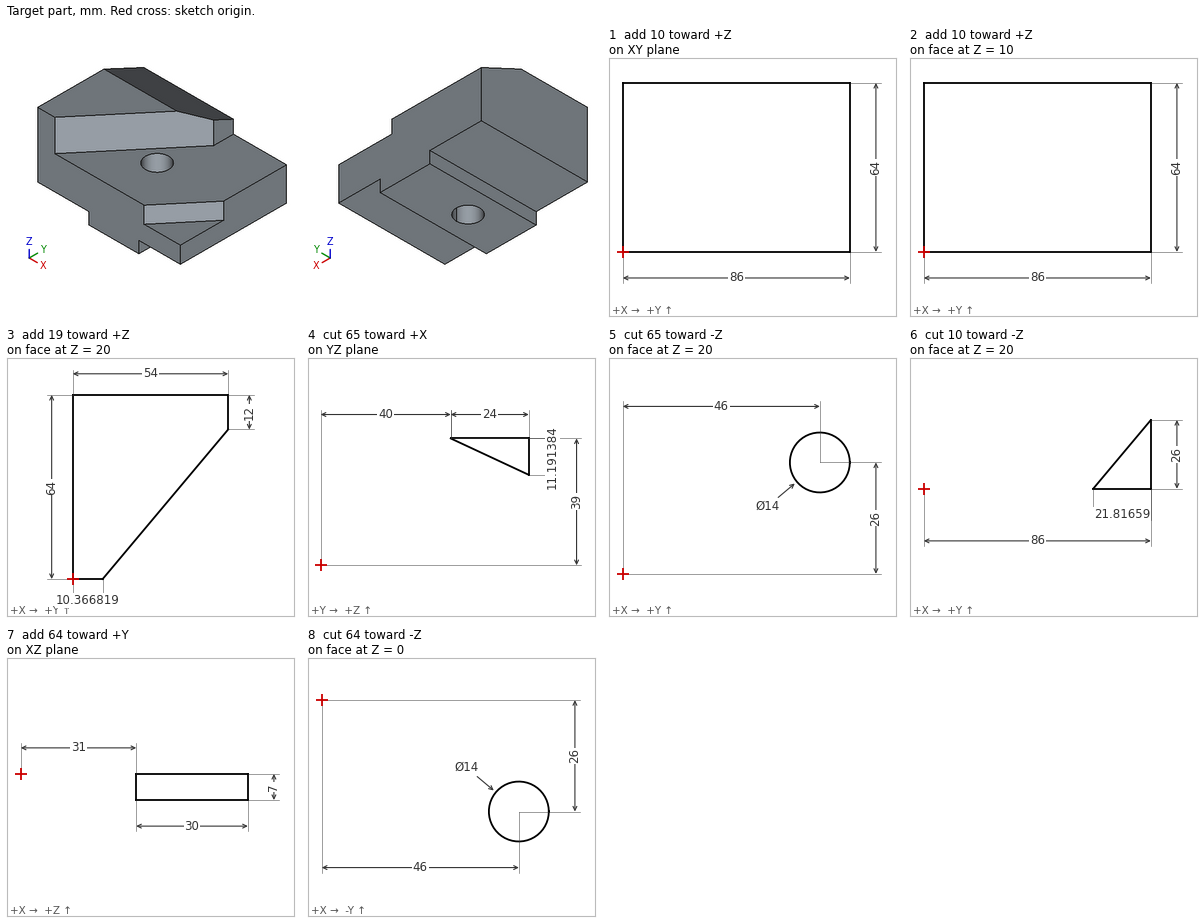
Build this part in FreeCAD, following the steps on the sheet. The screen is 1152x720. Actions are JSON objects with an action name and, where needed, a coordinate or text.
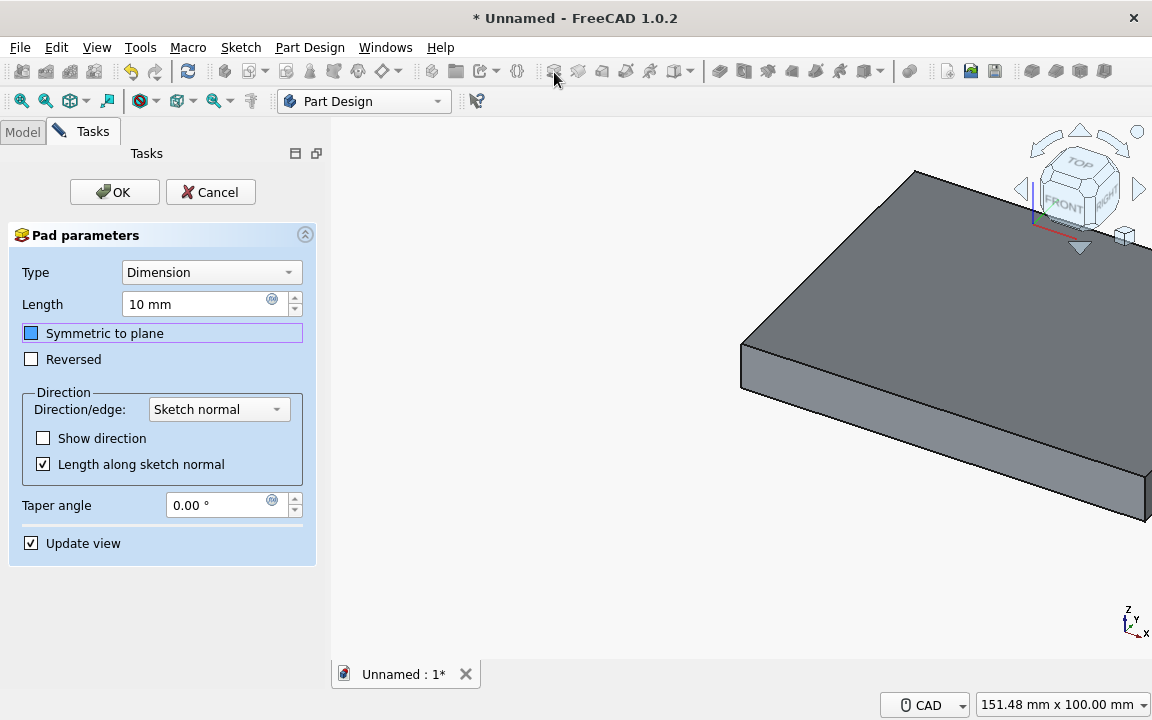
{"action": "left_click", "coordinate": [115, 192]}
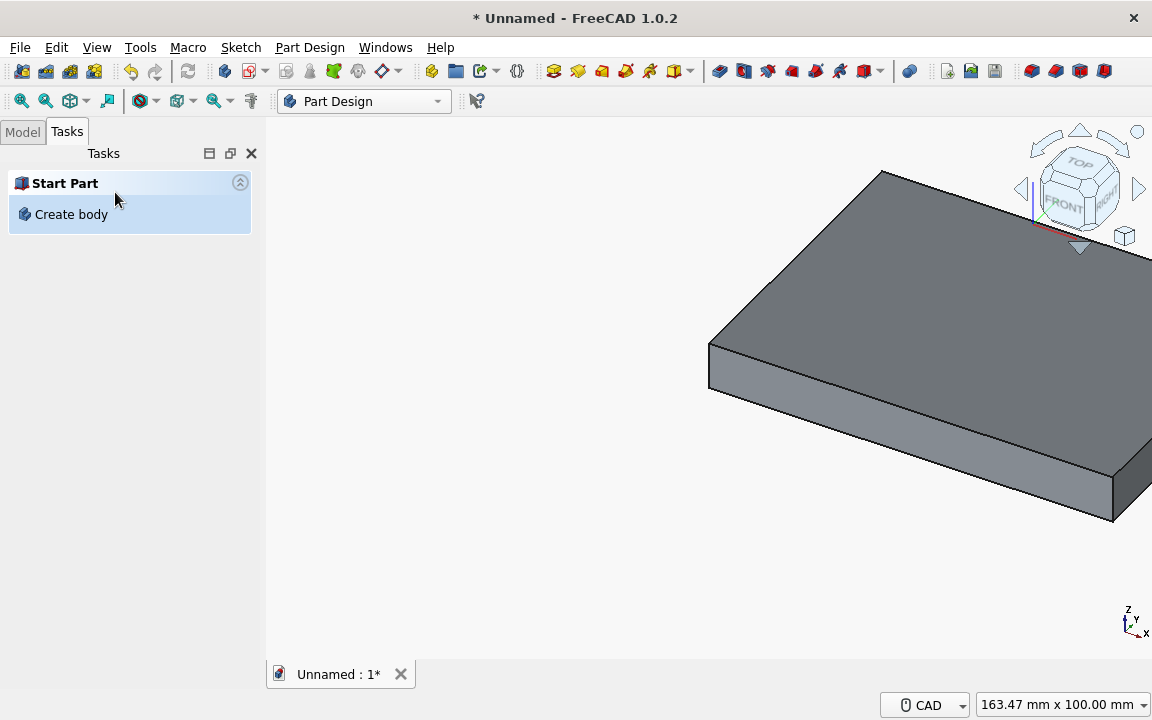
{"action": "left_click", "coordinate": [22, 102]}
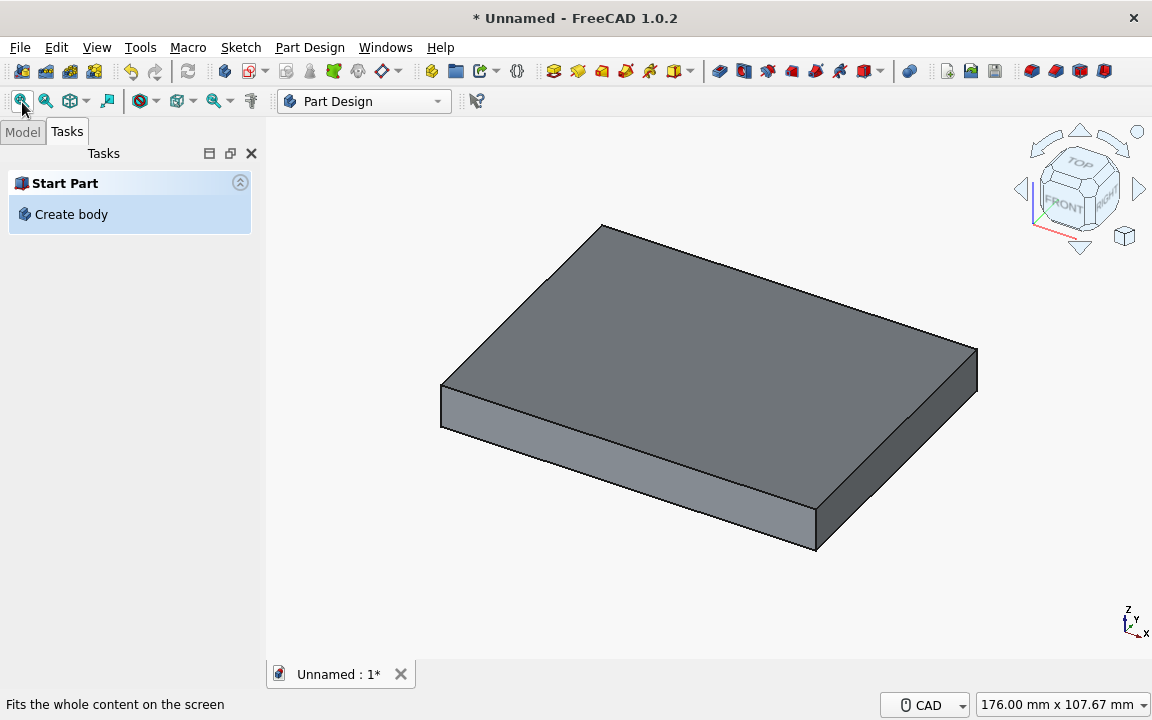
{"action": "left_click", "coordinate": [709, 366]}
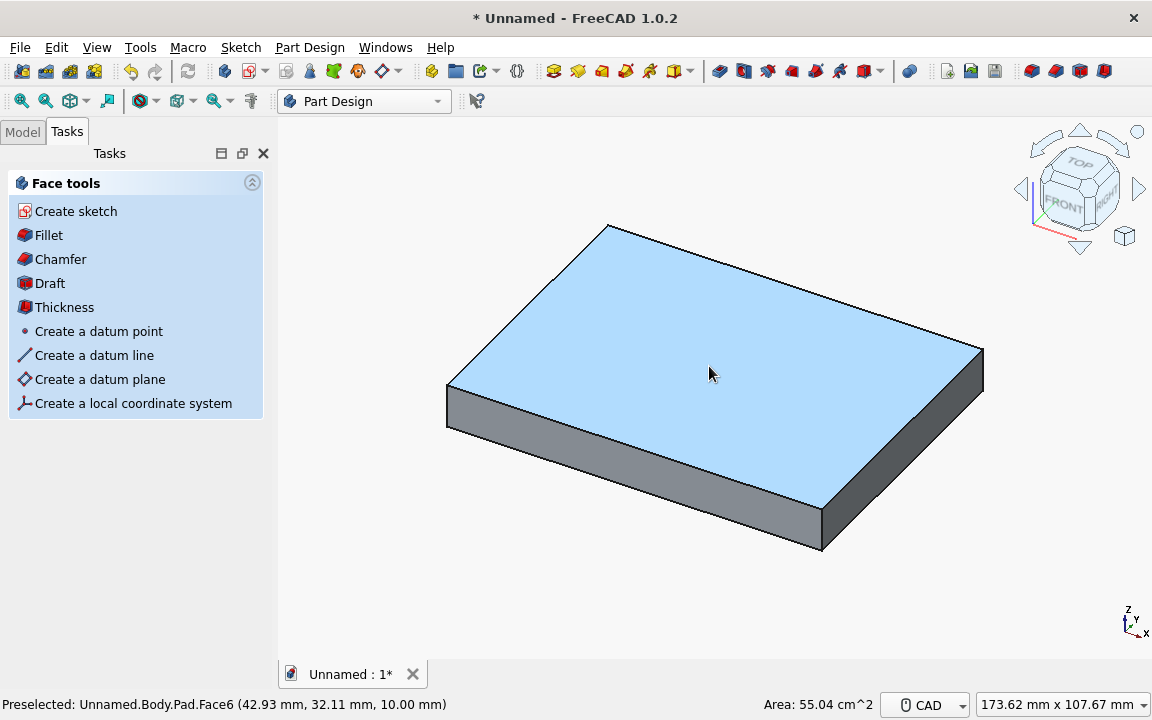
{"action": "left_click", "coordinate": [250, 72]}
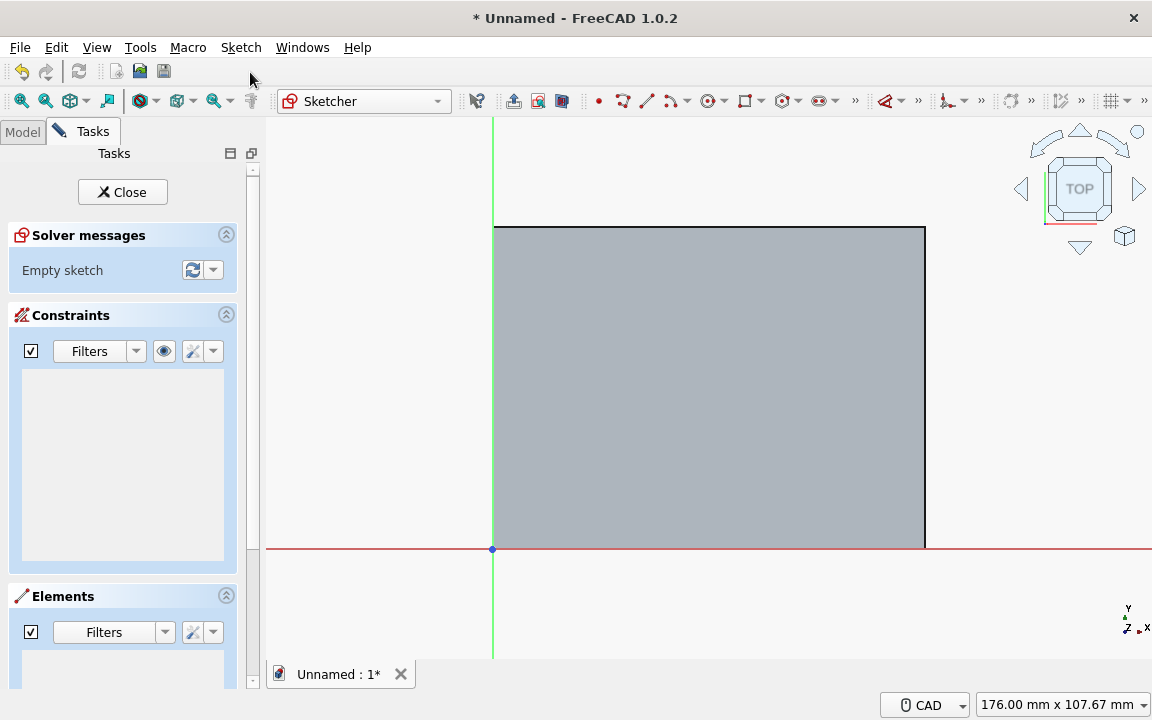
{"action": "left_click", "coordinate": [746, 102]}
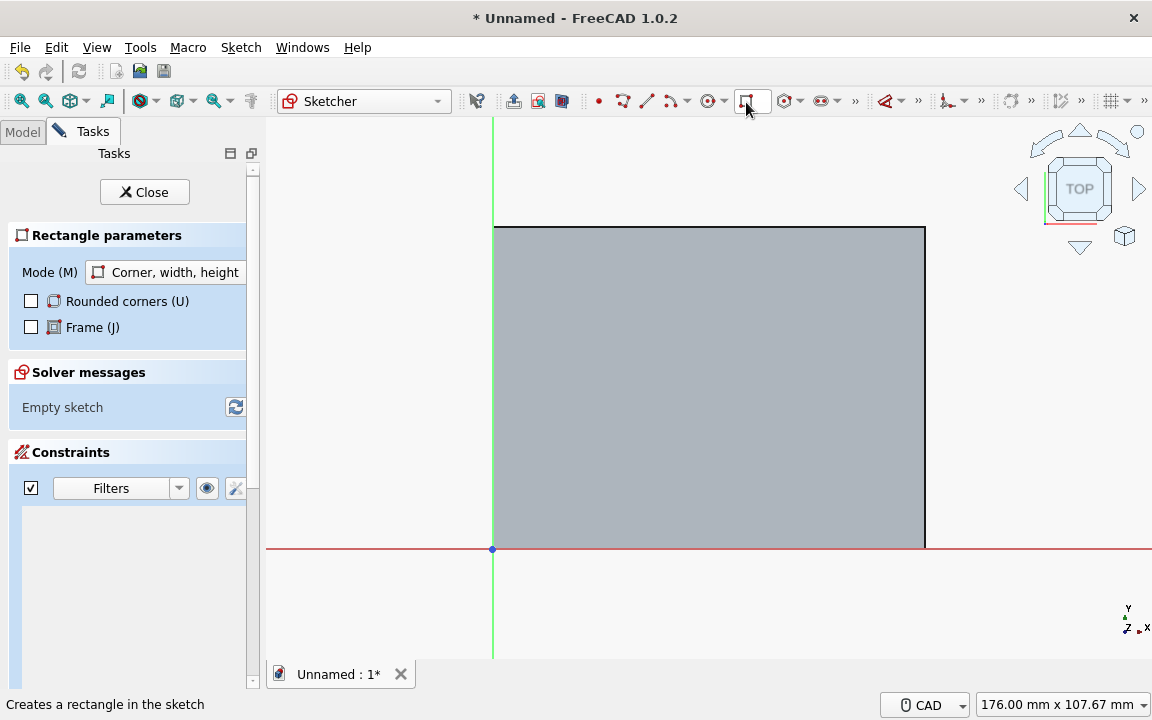
{"action": "left_click", "coordinate": [493, 549]}
{"action": "mouse_move", "coordinate": [925, 227]}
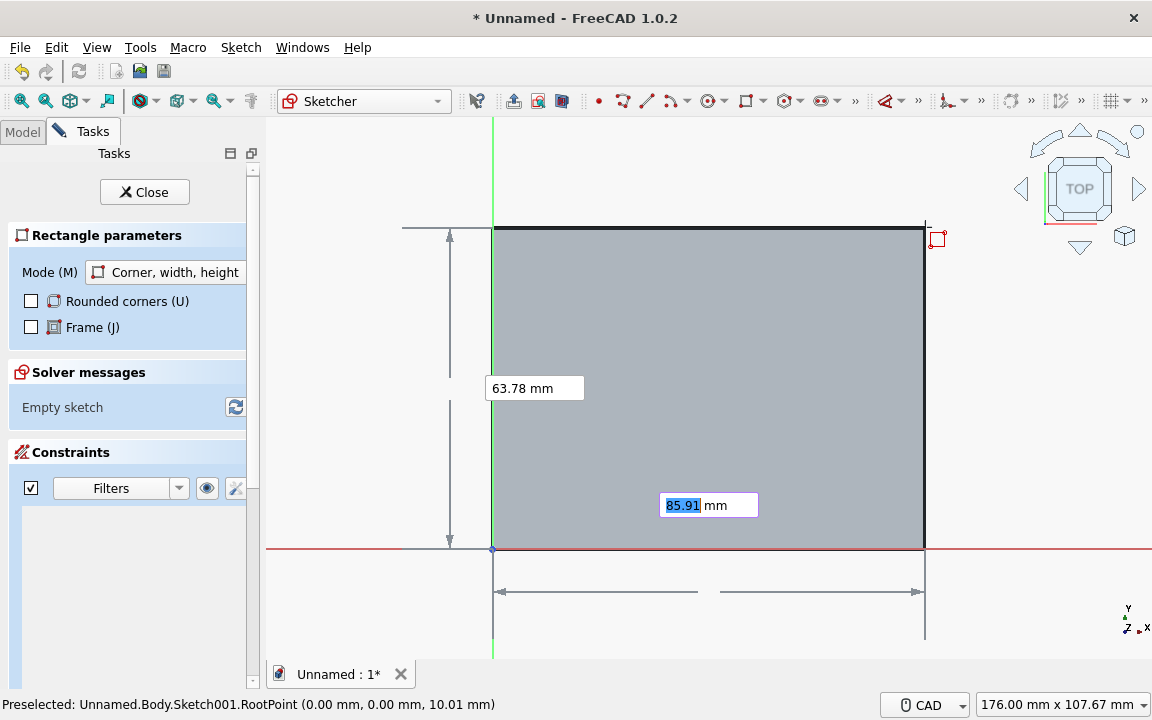
{"action": "type", "text": "86"}
{"action": "key", "text": "Tab"}
{"action": "type", "text": "64"}
{"action": "key", "text": "Return"}
{"action": "key", "text": "Escape"}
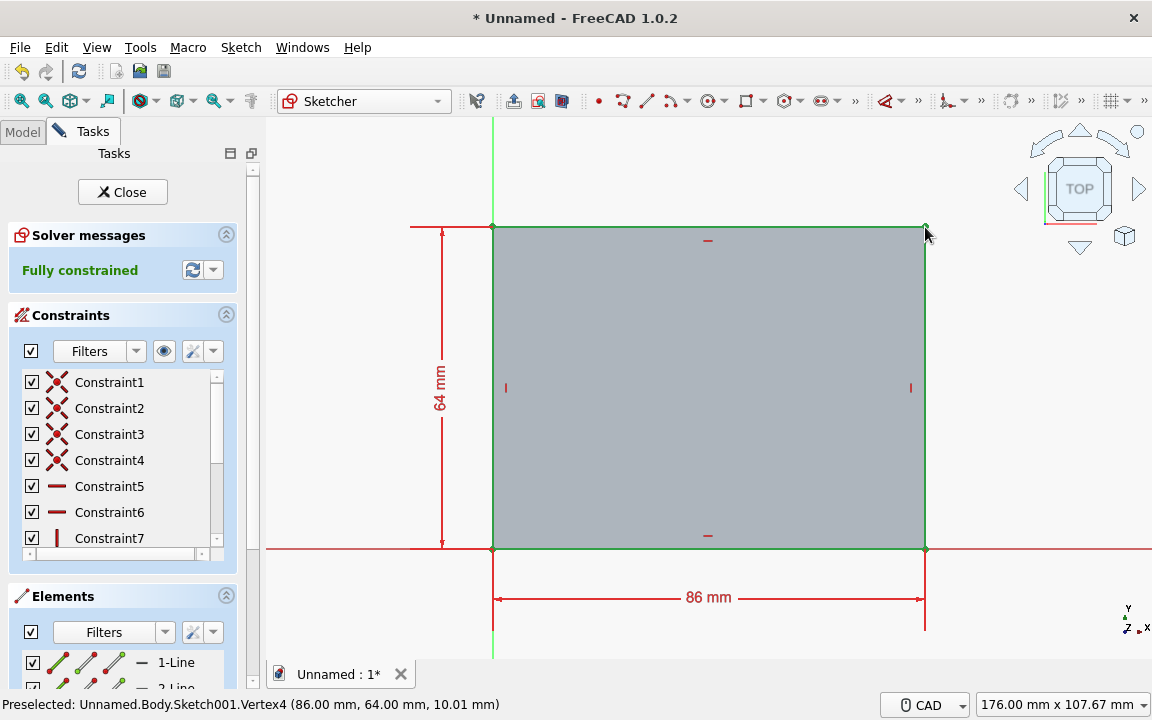
{"action": "left_click", "coordinate": [123, 192]}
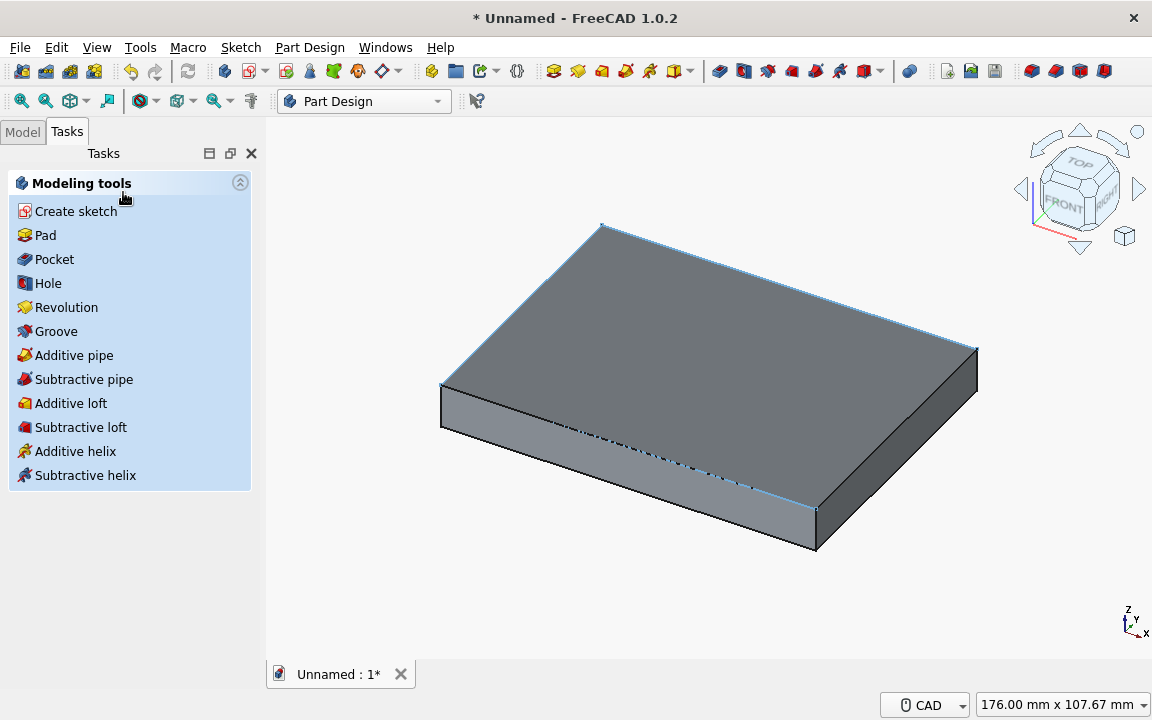
{"action": "left_click", "coordinate": [554, 72]}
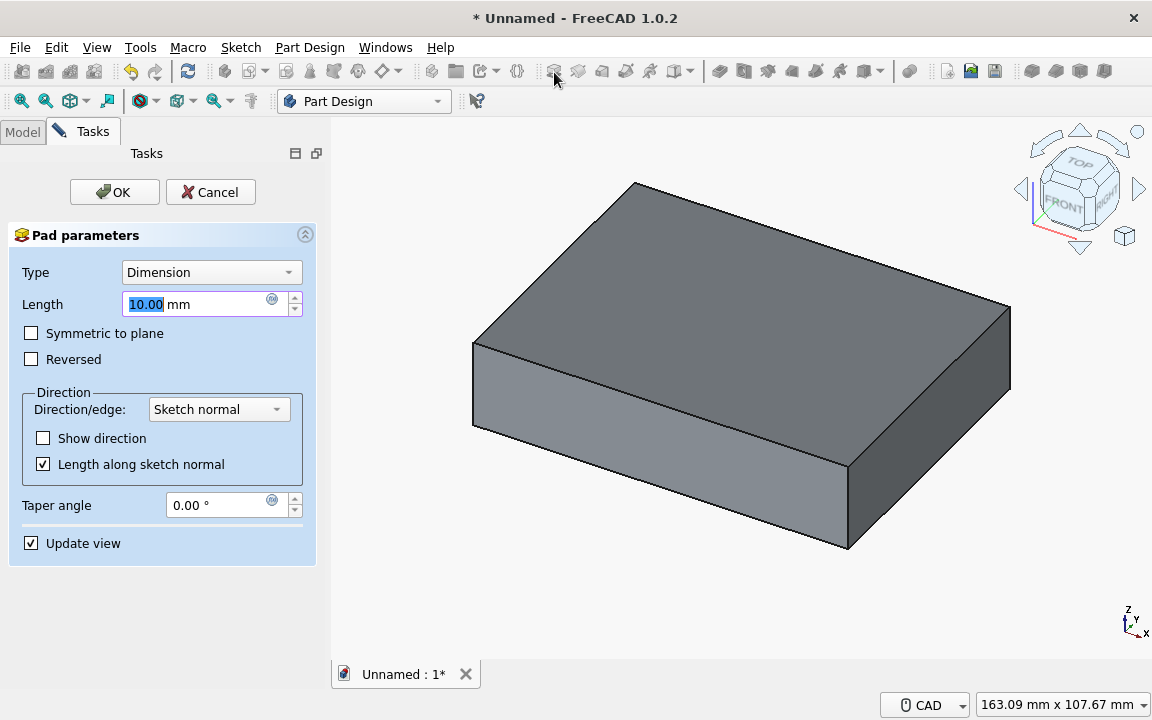
{"action": "type", "text": "10"}
{"action": "key", "text": "Tab"}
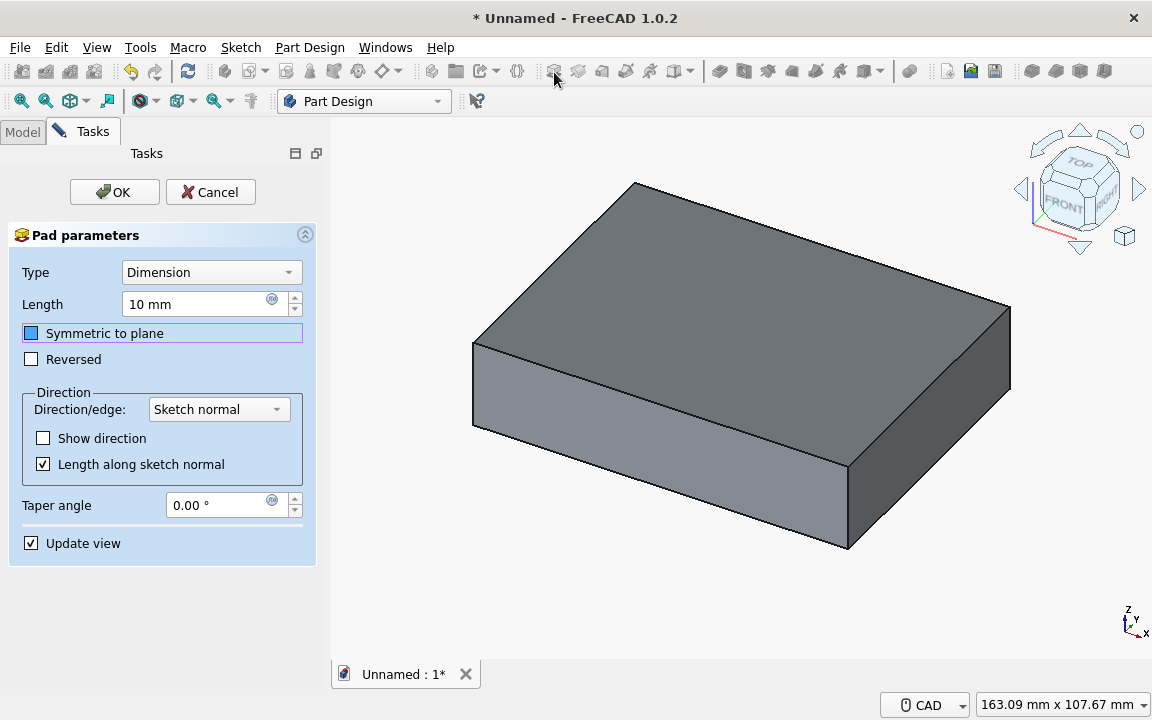
{"action": "left_click", "coordinate": [115, 192]}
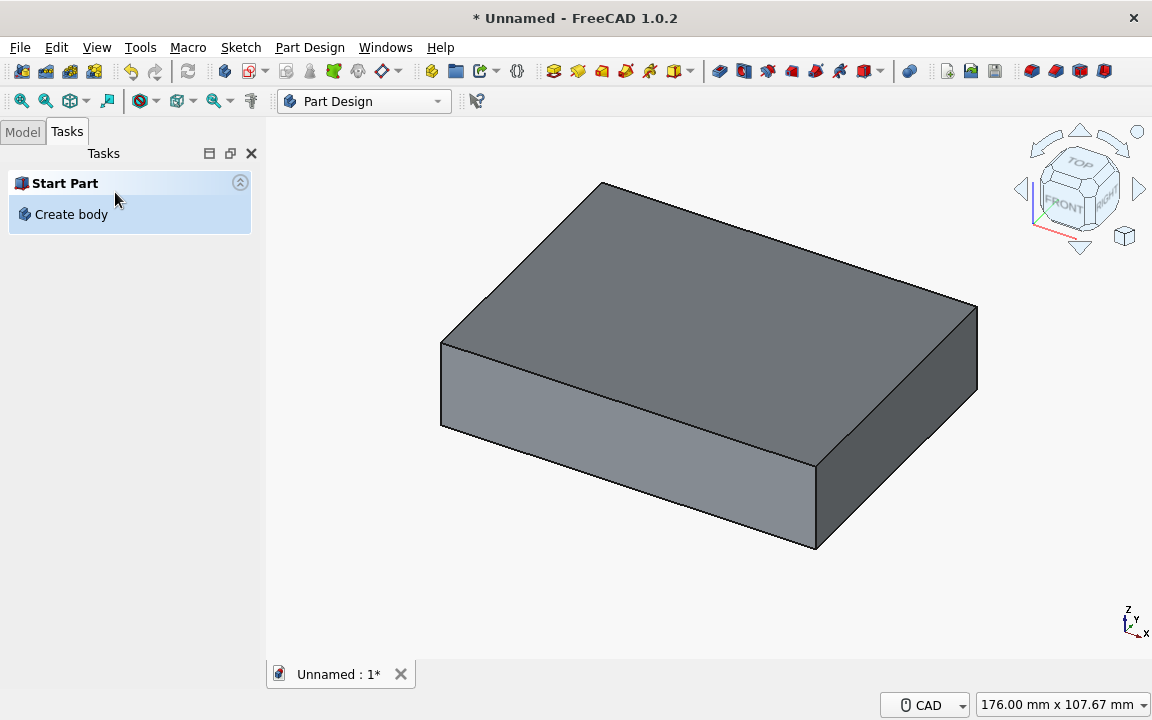
{"action": "left_click", "coordinate": [709, 324]}